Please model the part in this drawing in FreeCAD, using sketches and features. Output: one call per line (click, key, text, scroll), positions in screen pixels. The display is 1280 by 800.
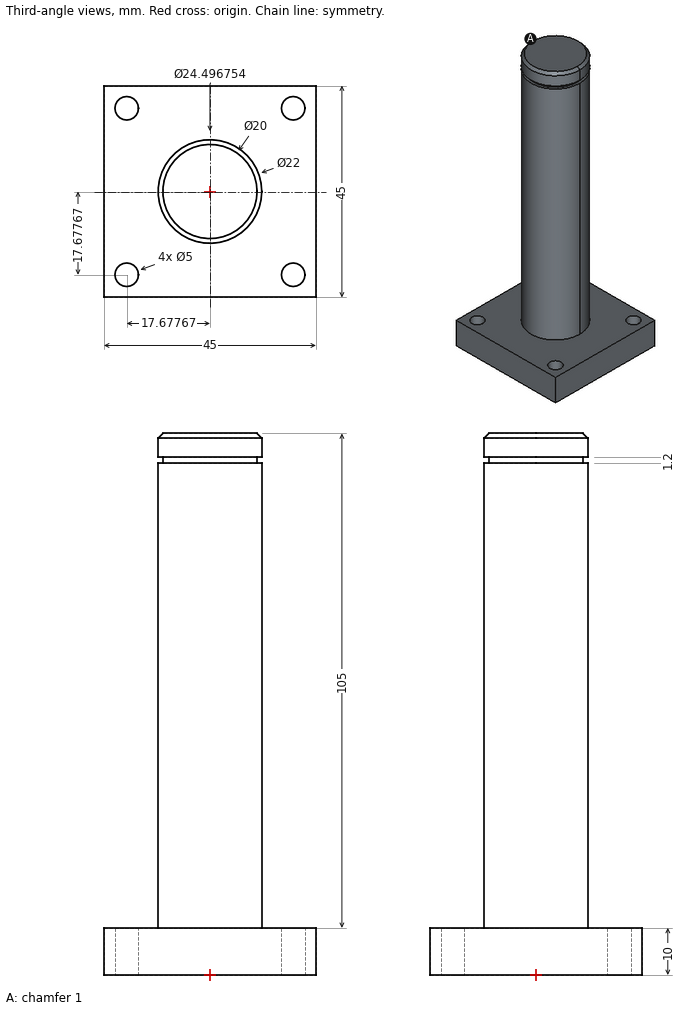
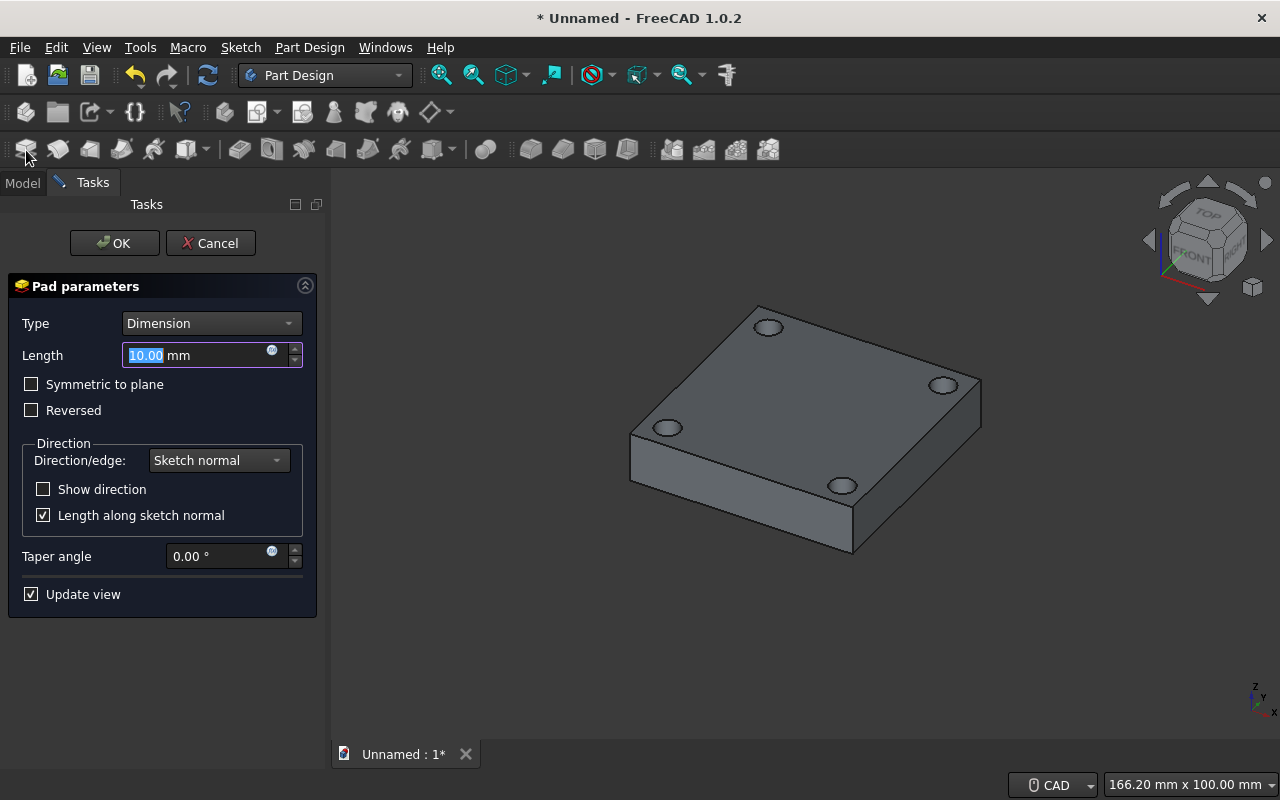
text(10)
key(Tab)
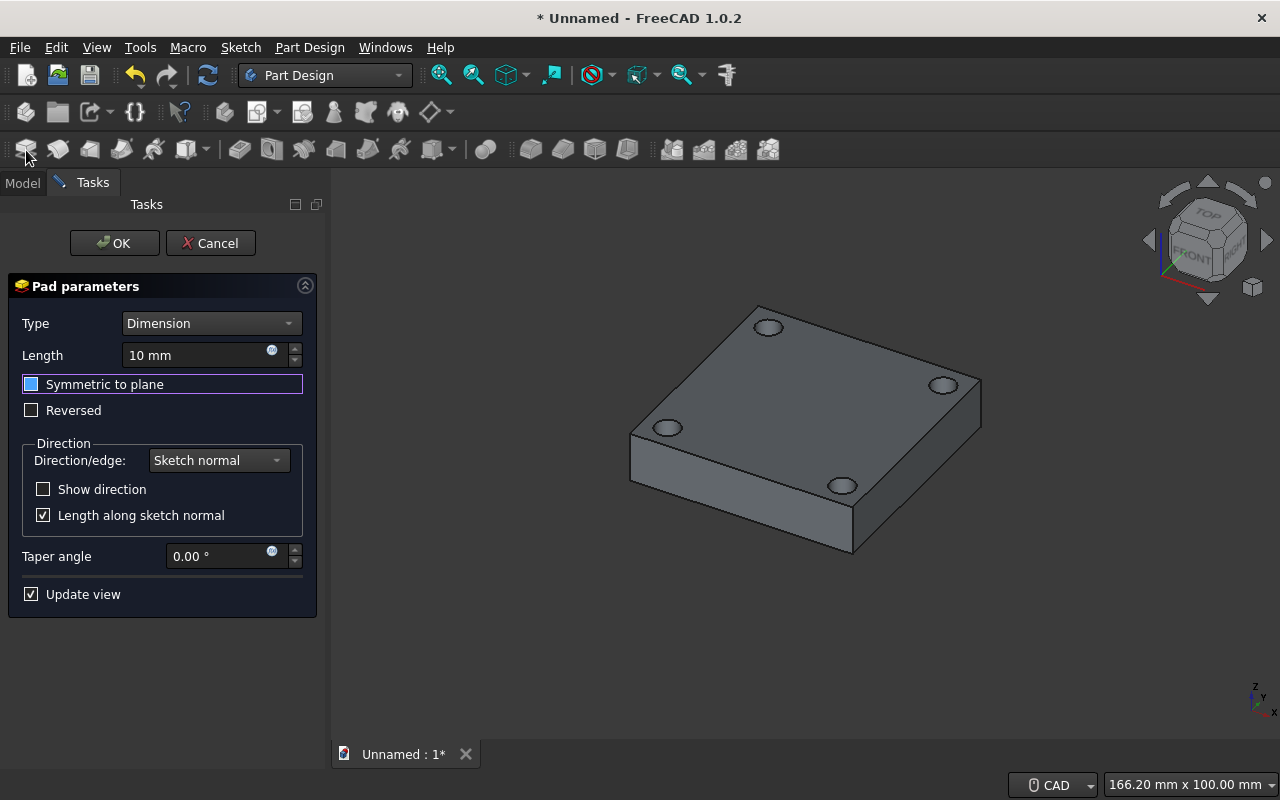
click(115, 243)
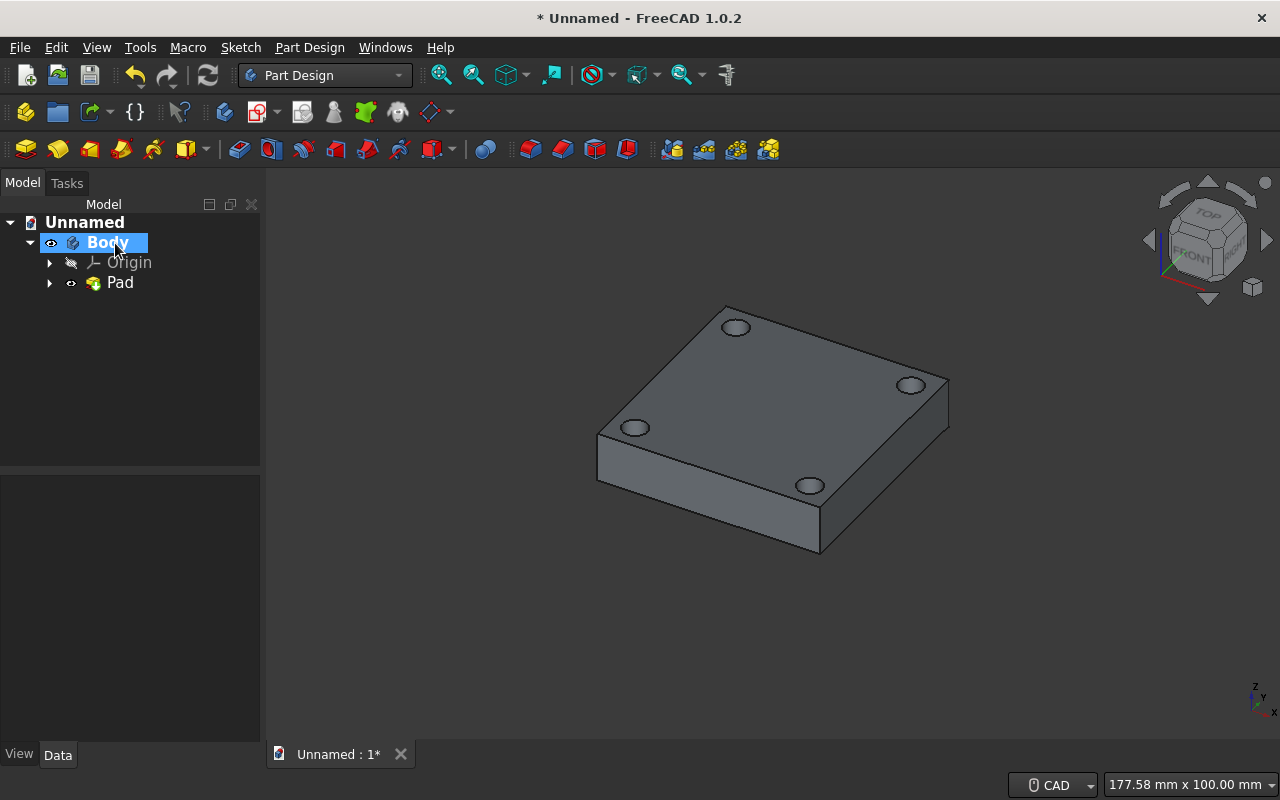
click(442, 76)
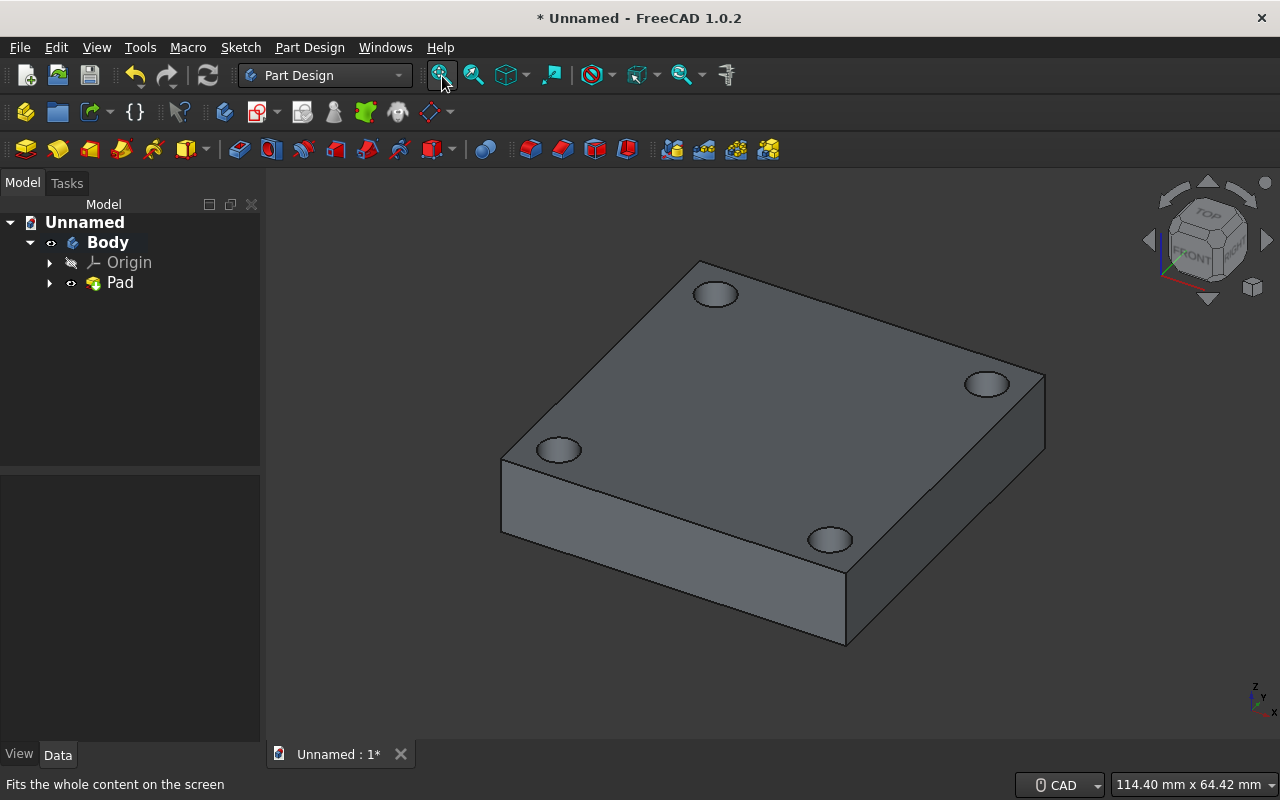
click(773, 416)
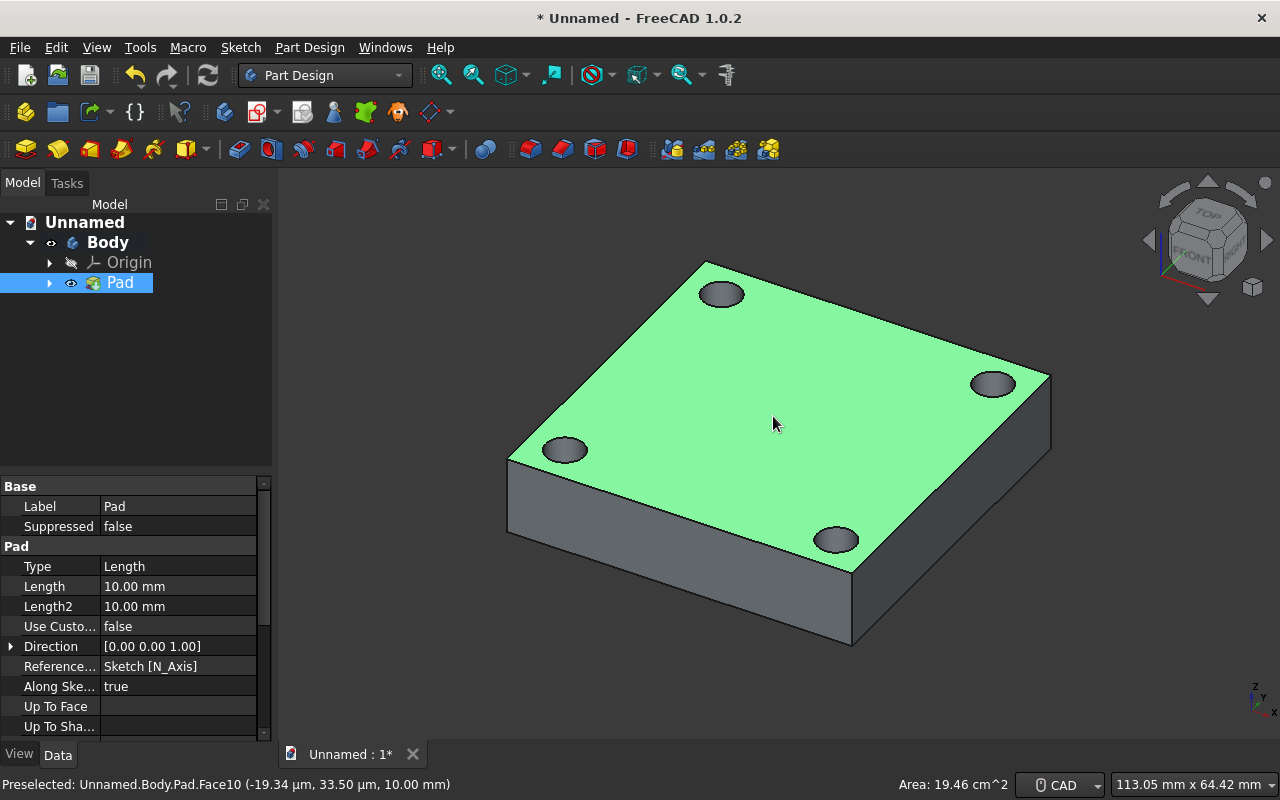
click(258, 112)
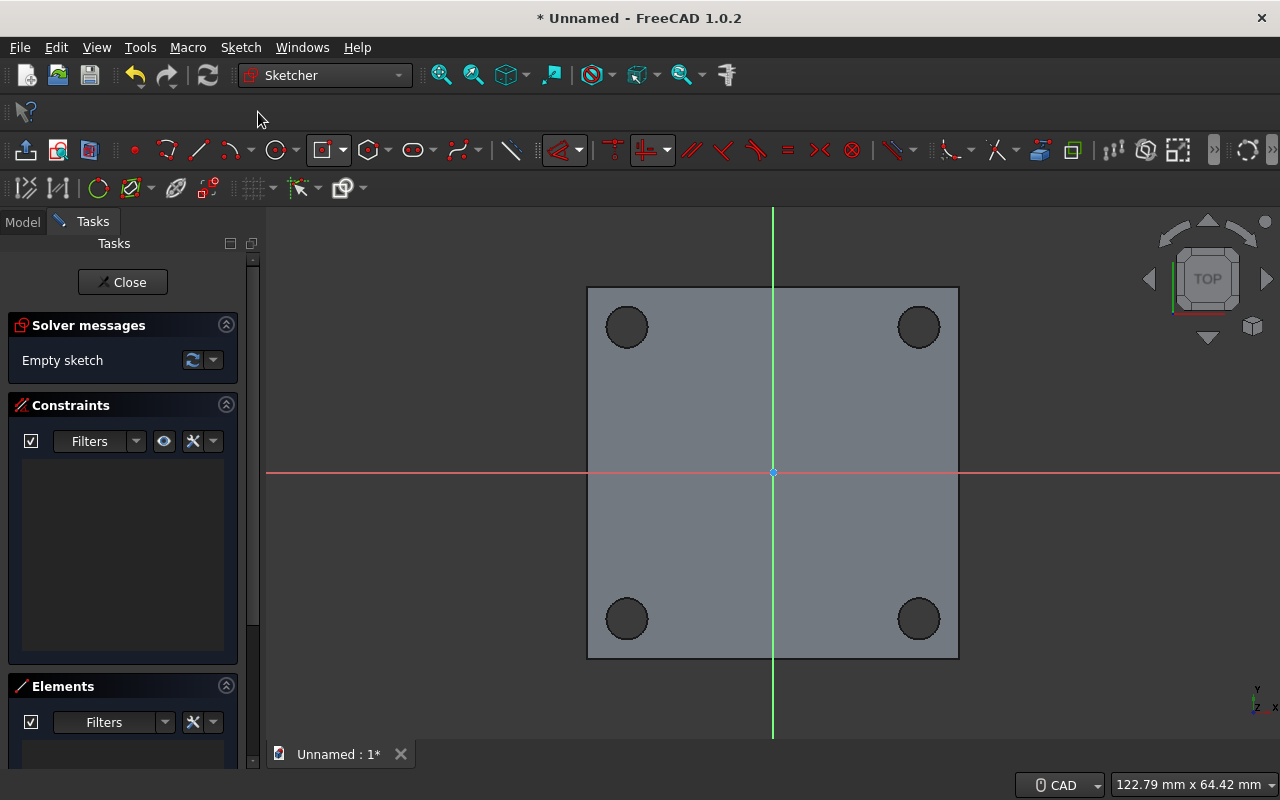
scroll(856, 473, up, 3)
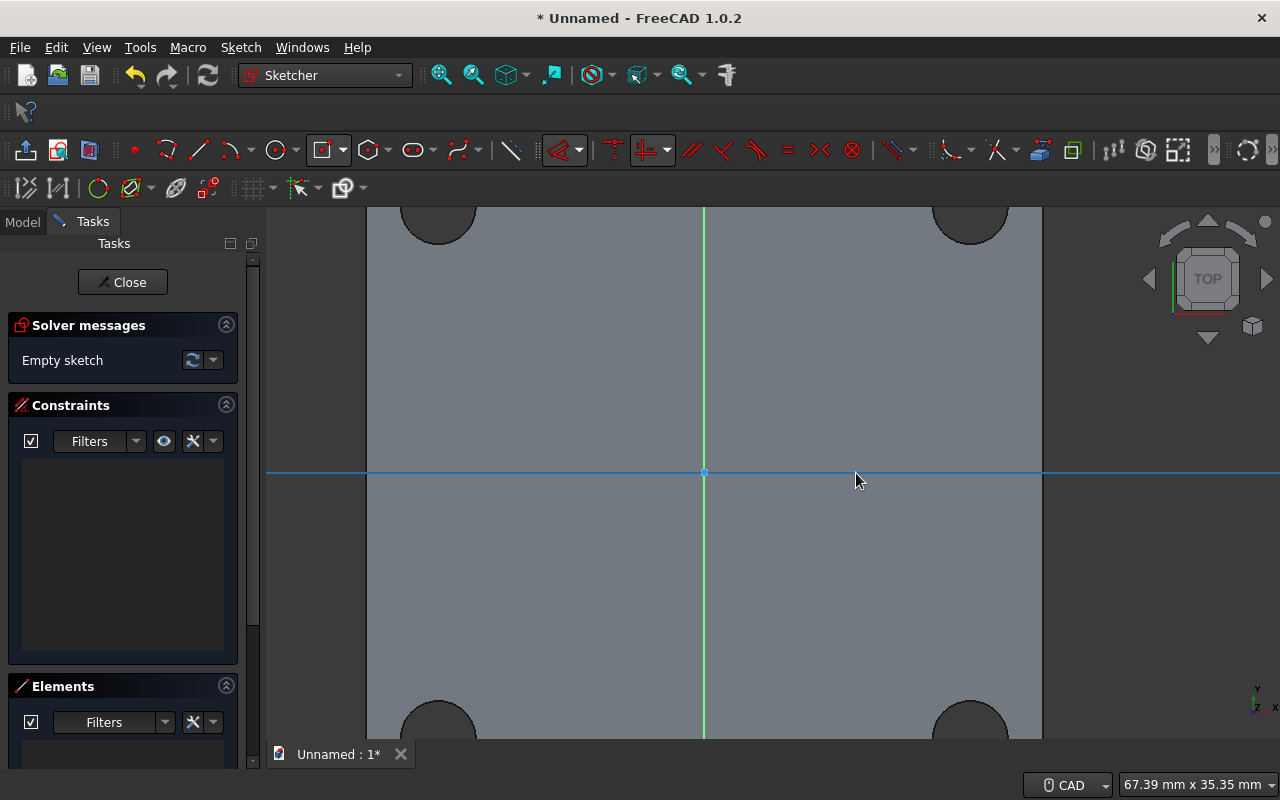
click(276, 150)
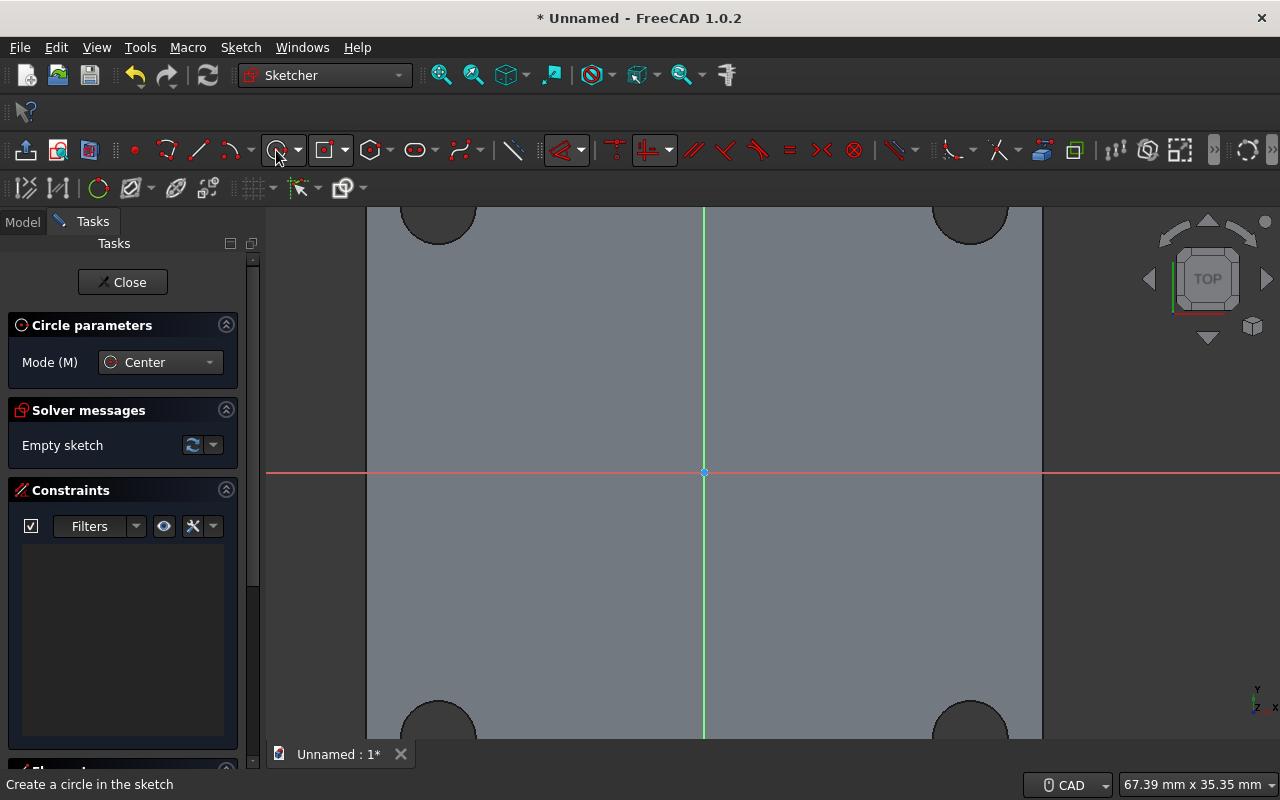
click(704, 473)
move(821, 356)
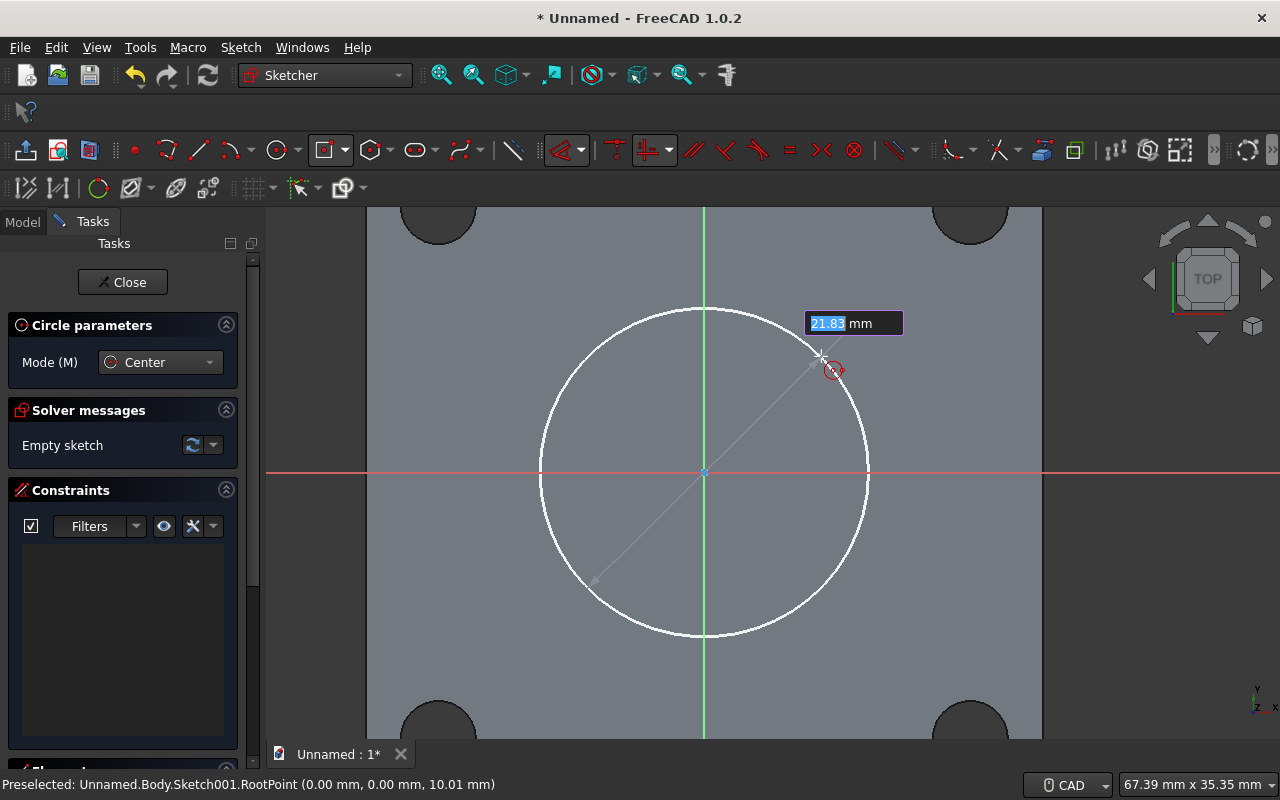
text(22)
key(Return)
key(Escape)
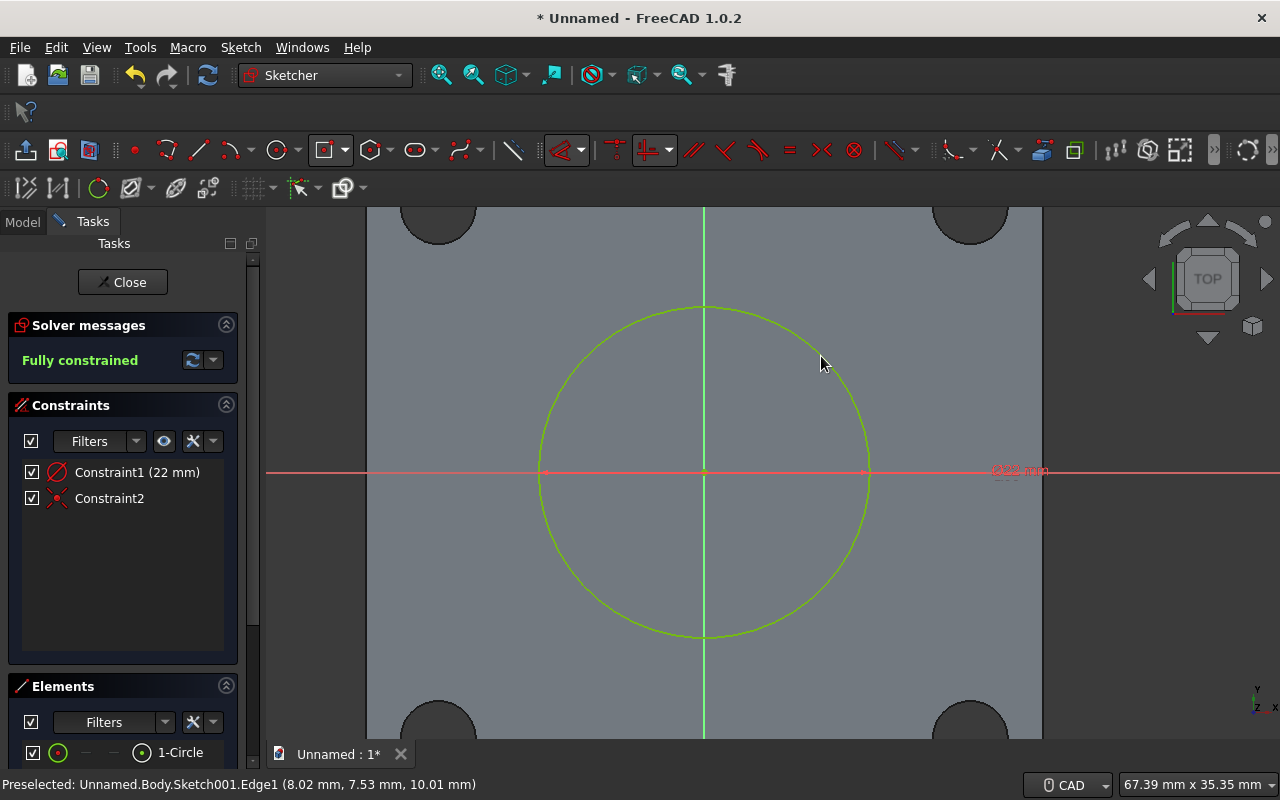
click(123, 282)